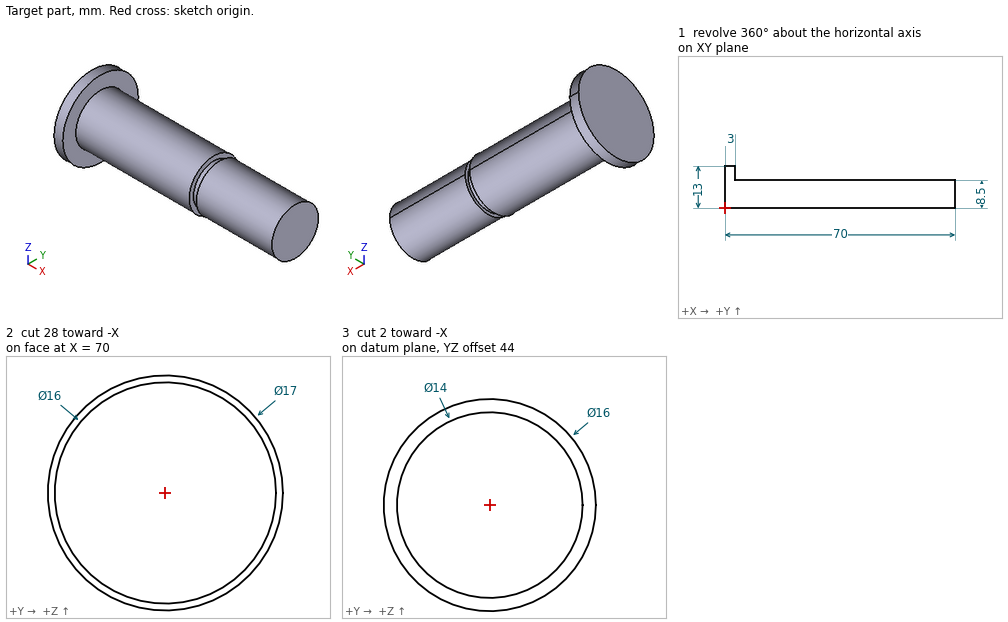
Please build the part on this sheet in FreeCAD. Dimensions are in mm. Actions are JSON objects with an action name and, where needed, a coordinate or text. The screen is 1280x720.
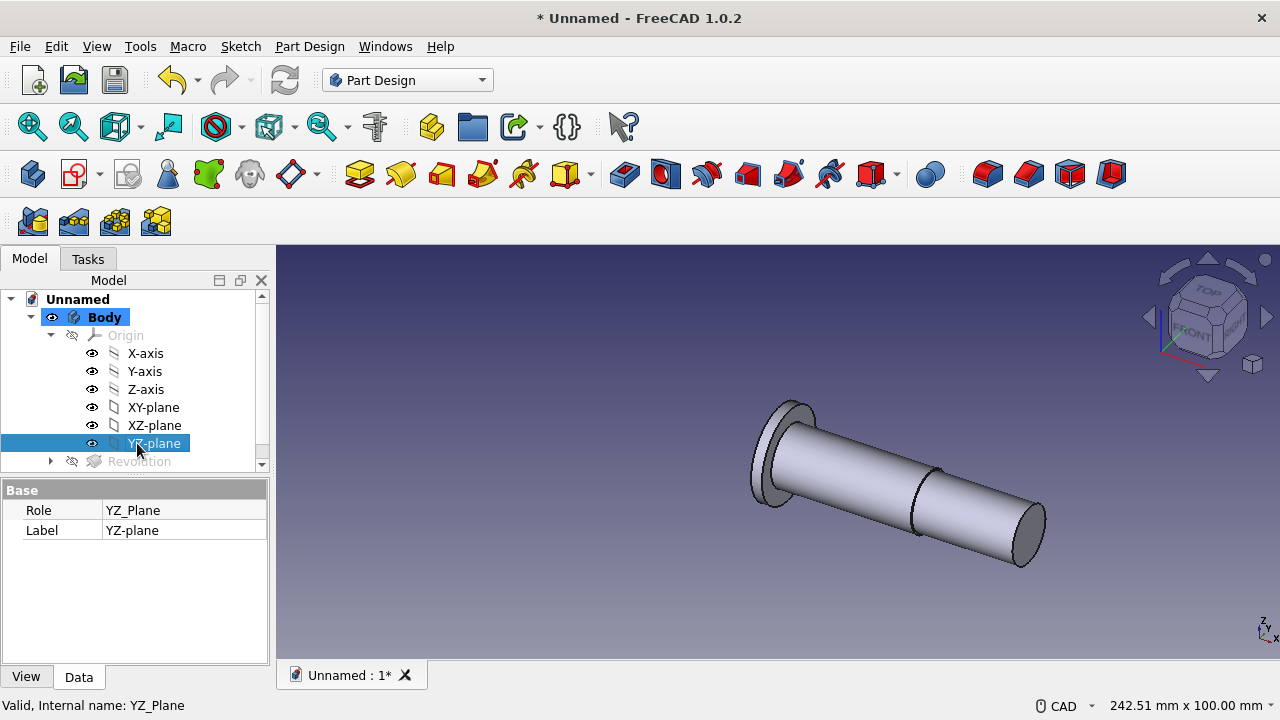
{"action": "left_click", "coordinate": [290, 174]}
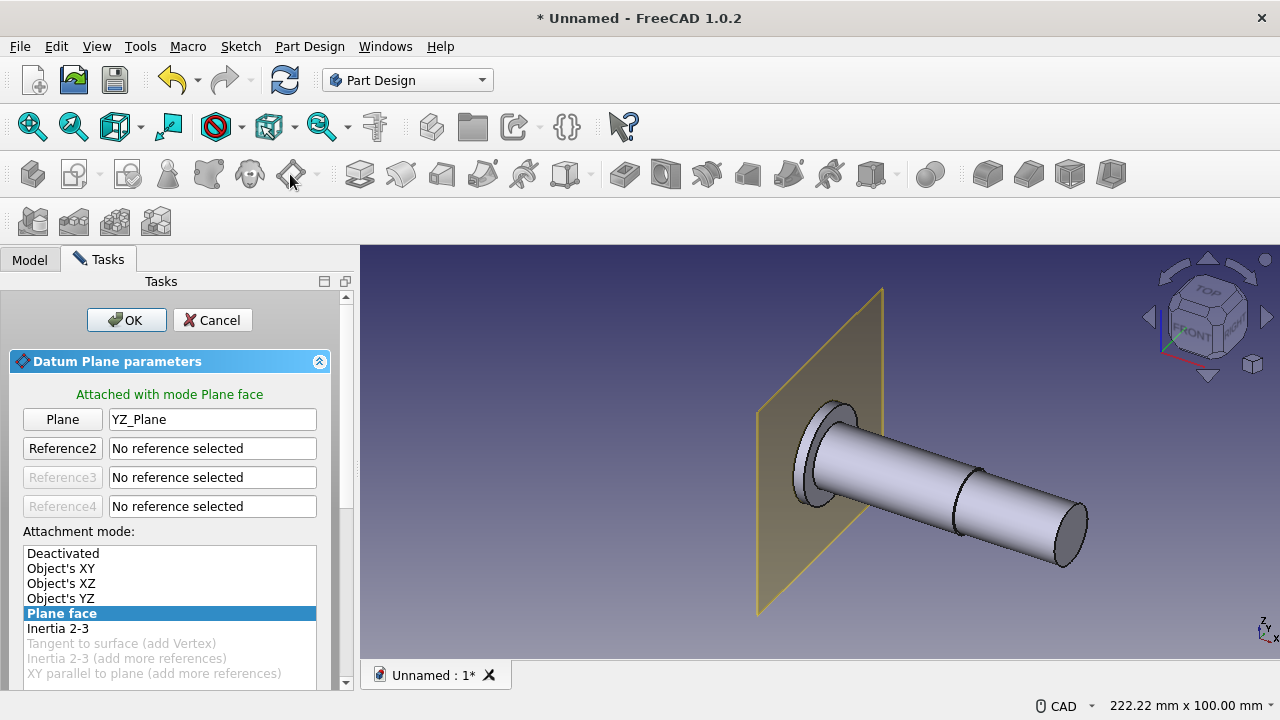
{"action": "scroll", "coordinate": [346, 490], "scroll_direction": "down", "scroll_amount": 4}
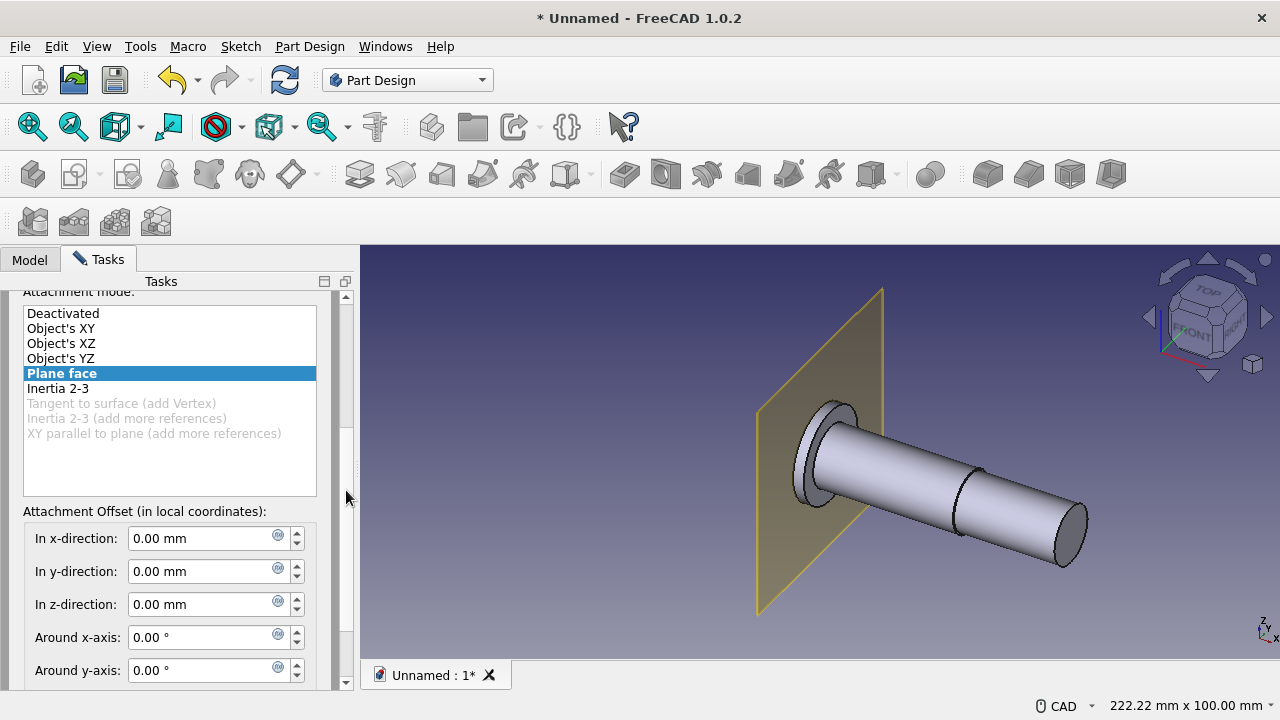
{"action": "triple_click", "coordinate": [210, 604]}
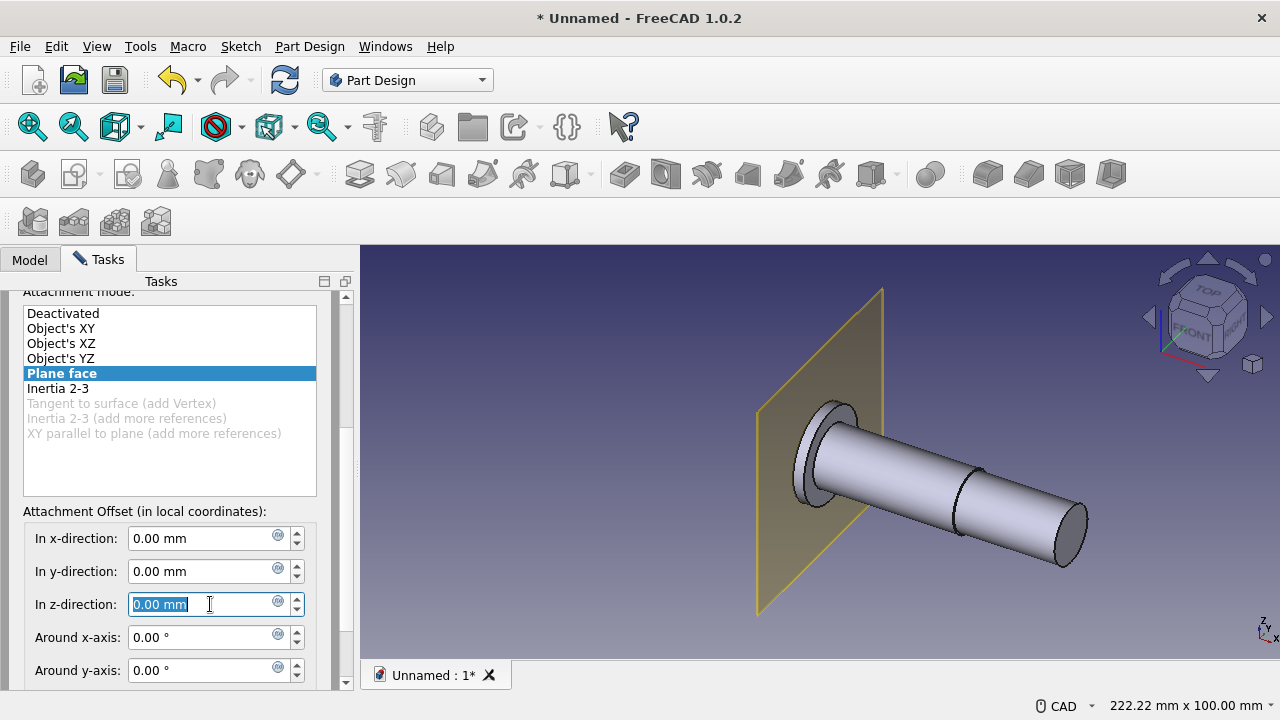
{"action": "type", "text": "44"}
{"action": "key", "text": "Tab"}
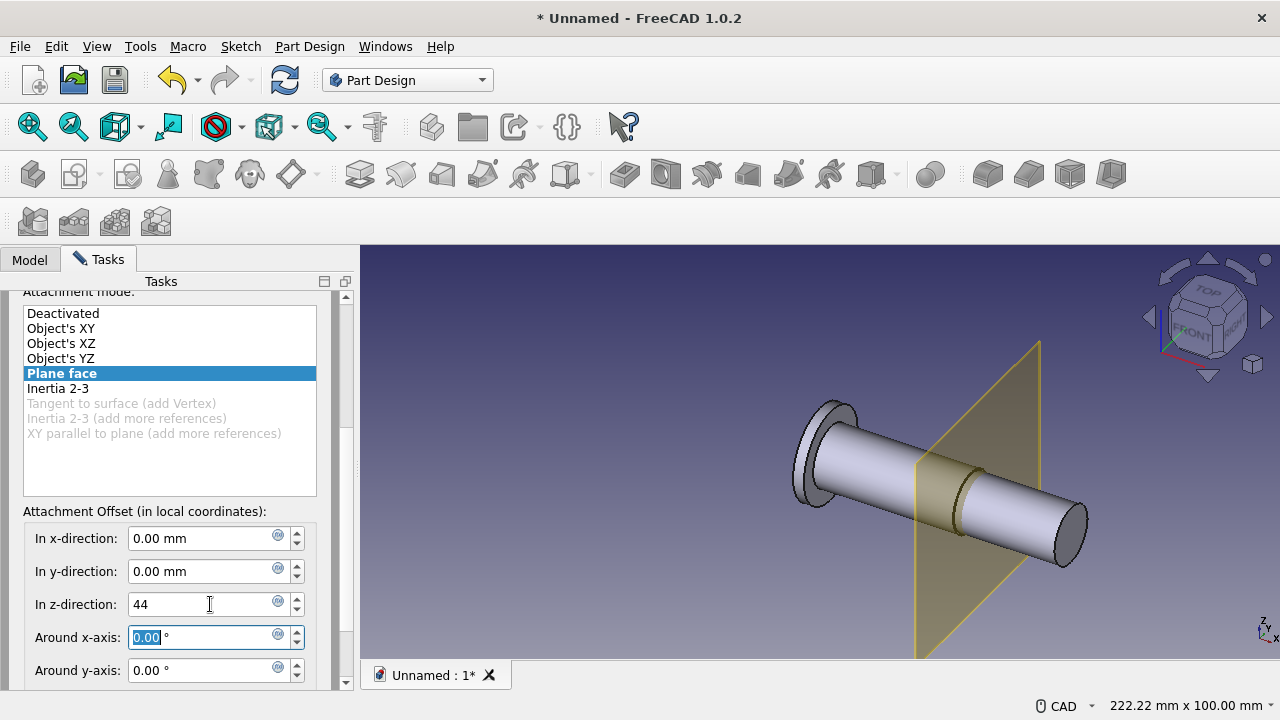
{"action": "scroll", "coordinate": [346, 490], "scroll_direction": "up", "scroll_amount": 5}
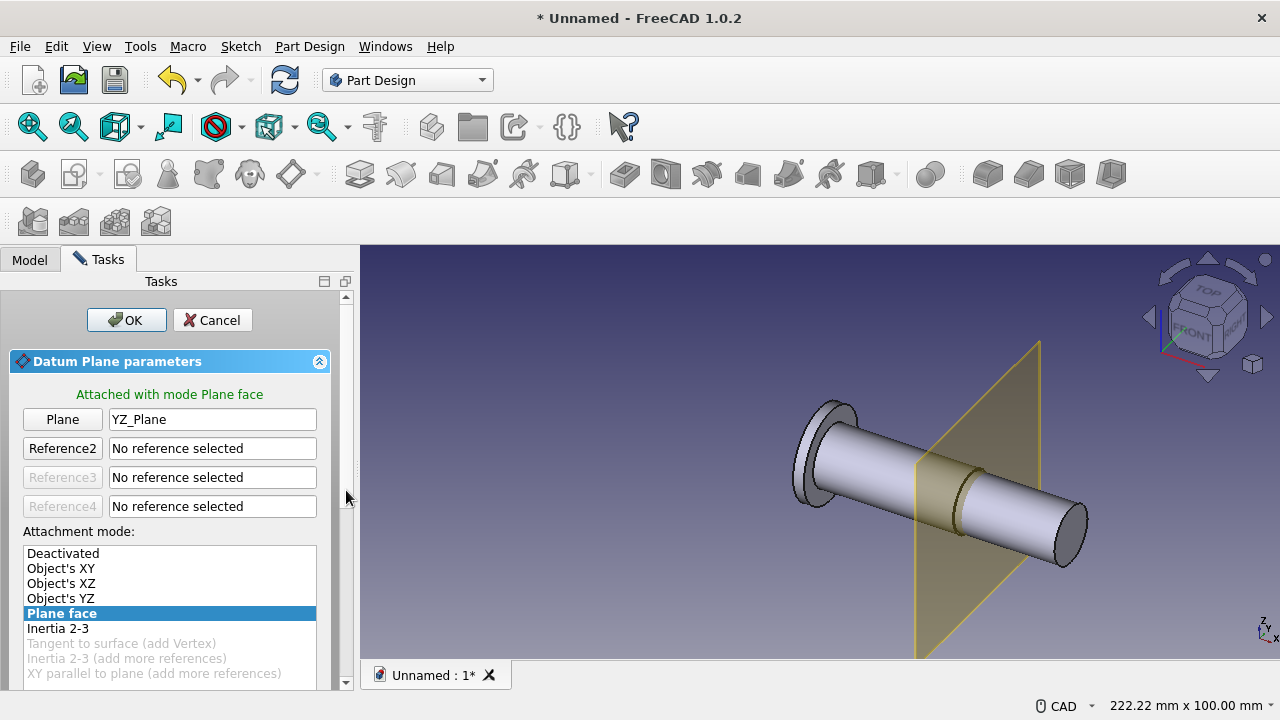
{"action": "left_click", "coordinate": [127, 320]}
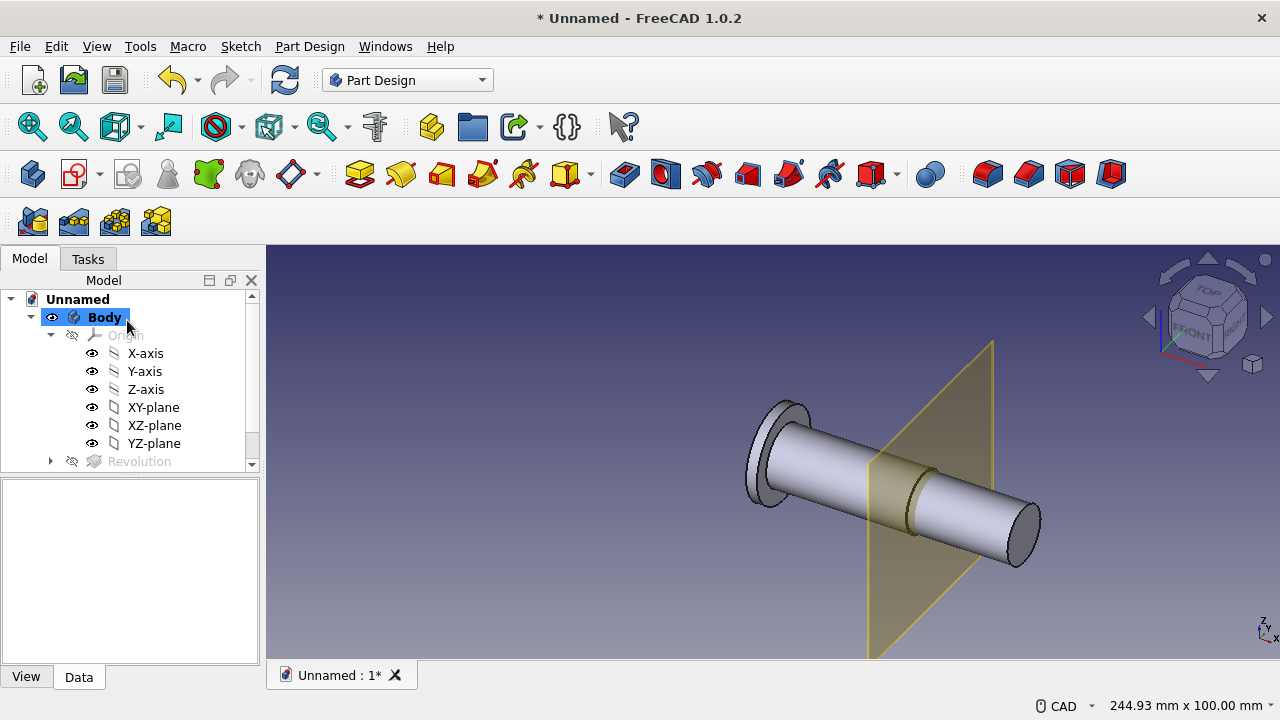
{"action": "scroll", "coordinate": [101, 385], "scroll_direction": "down", "scroll_amount": 3}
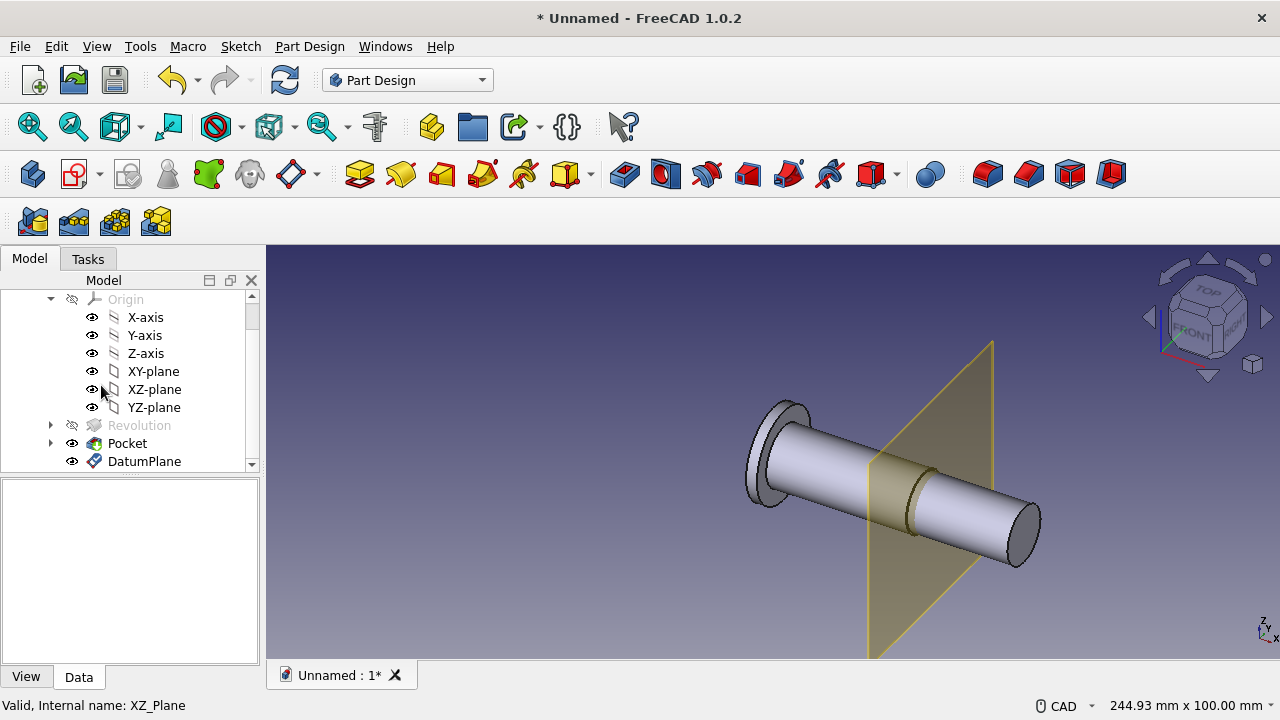
{"action": "left_click", "coordinate": [117, 461]}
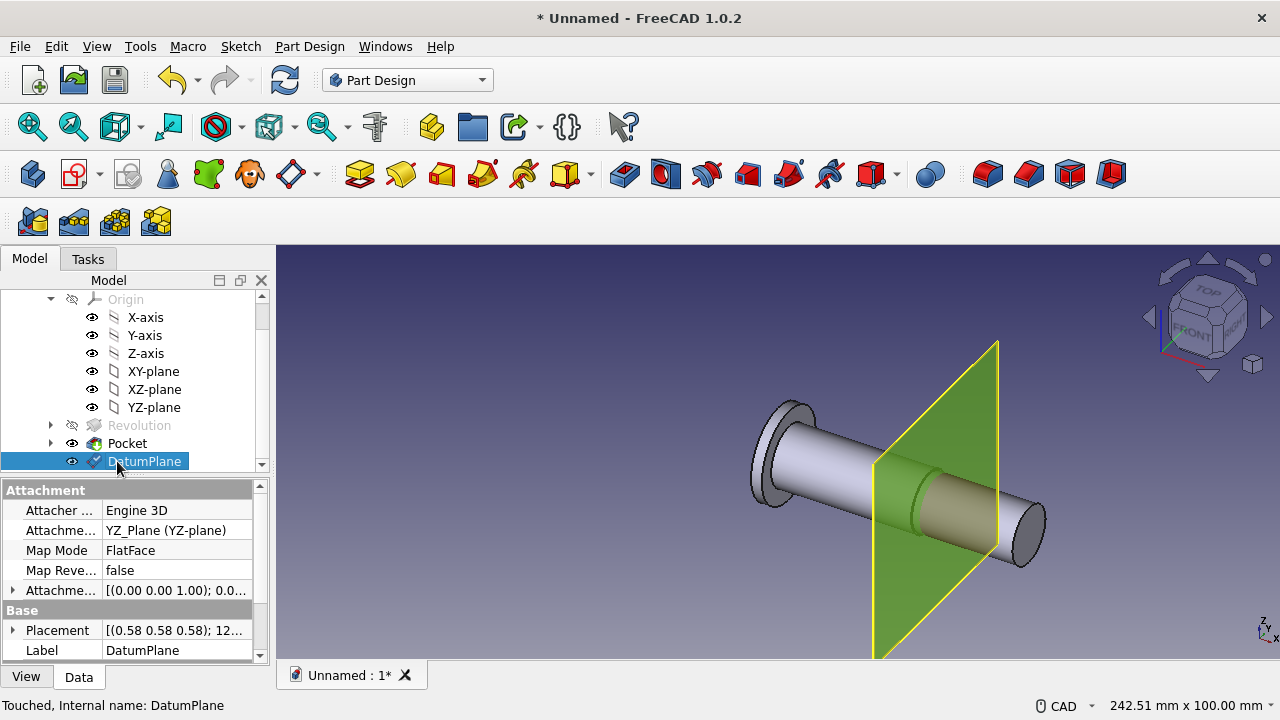
{"action": "left_click", "coordinate": [74, 174]}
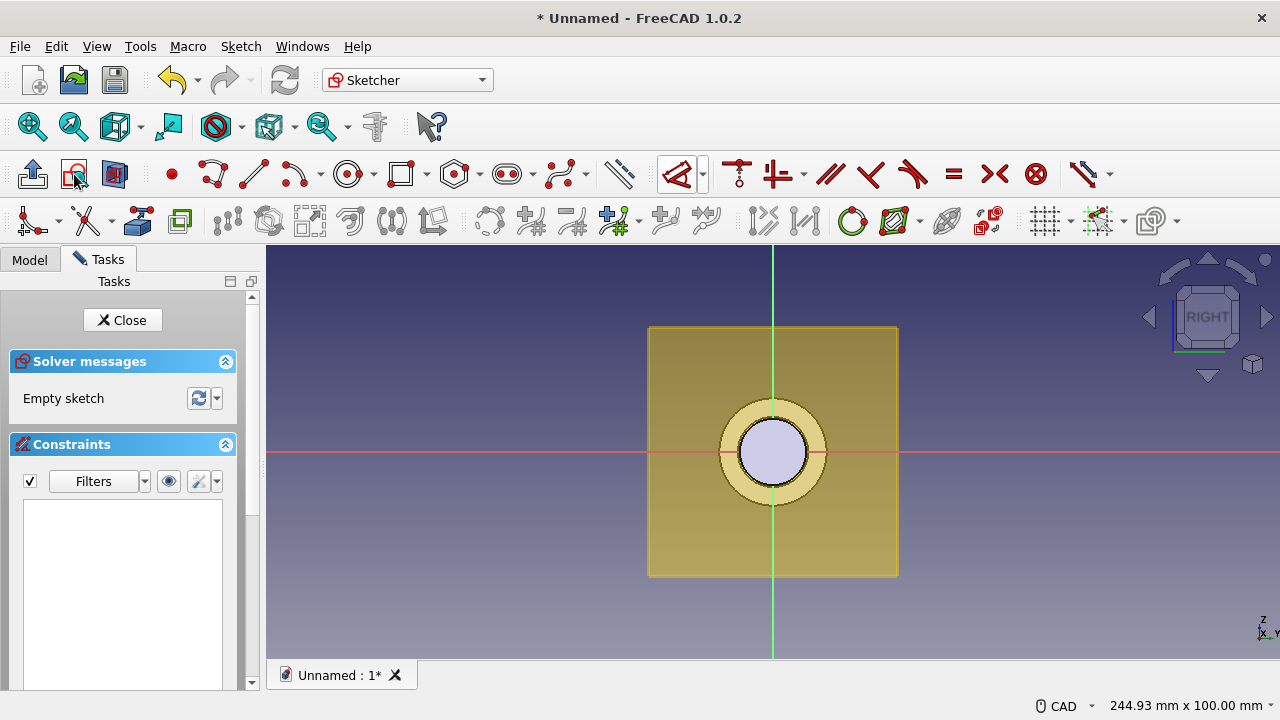
{"action": "key", "text": "q s"}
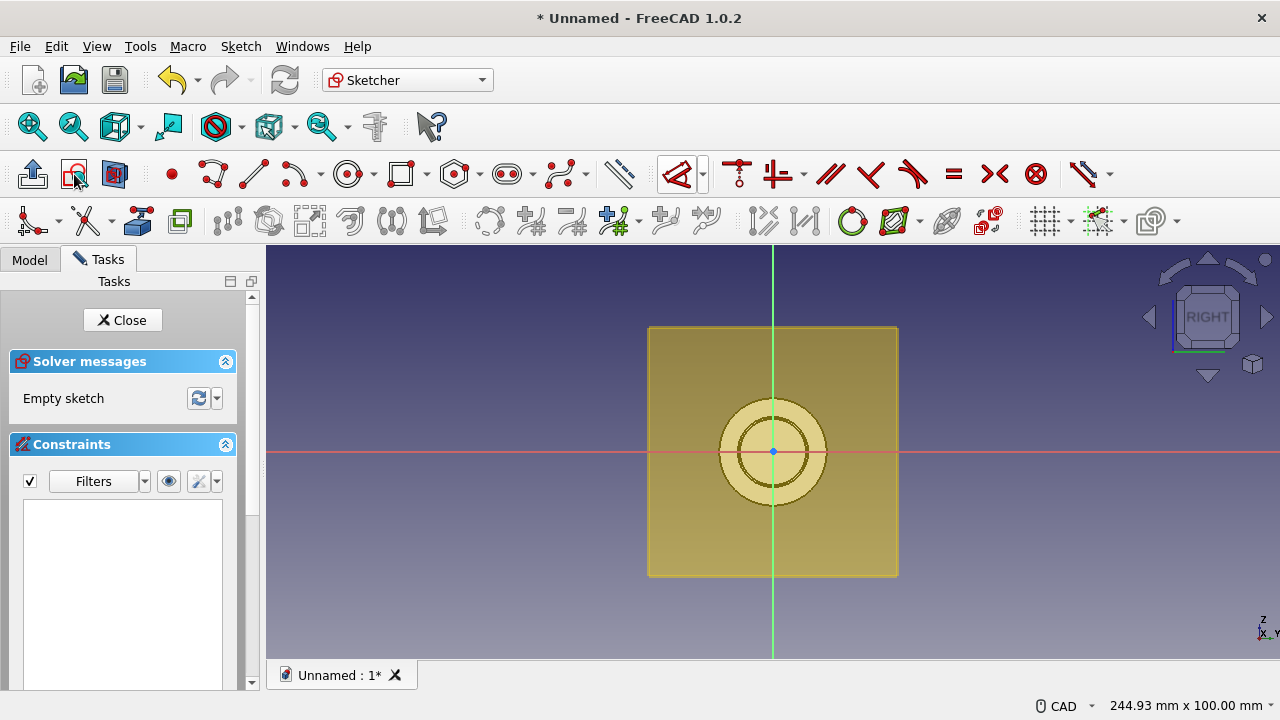
{"action": "scroll", "coordinate": [795, 452], "scroll_direction": "up", "scroll_amount": 7}